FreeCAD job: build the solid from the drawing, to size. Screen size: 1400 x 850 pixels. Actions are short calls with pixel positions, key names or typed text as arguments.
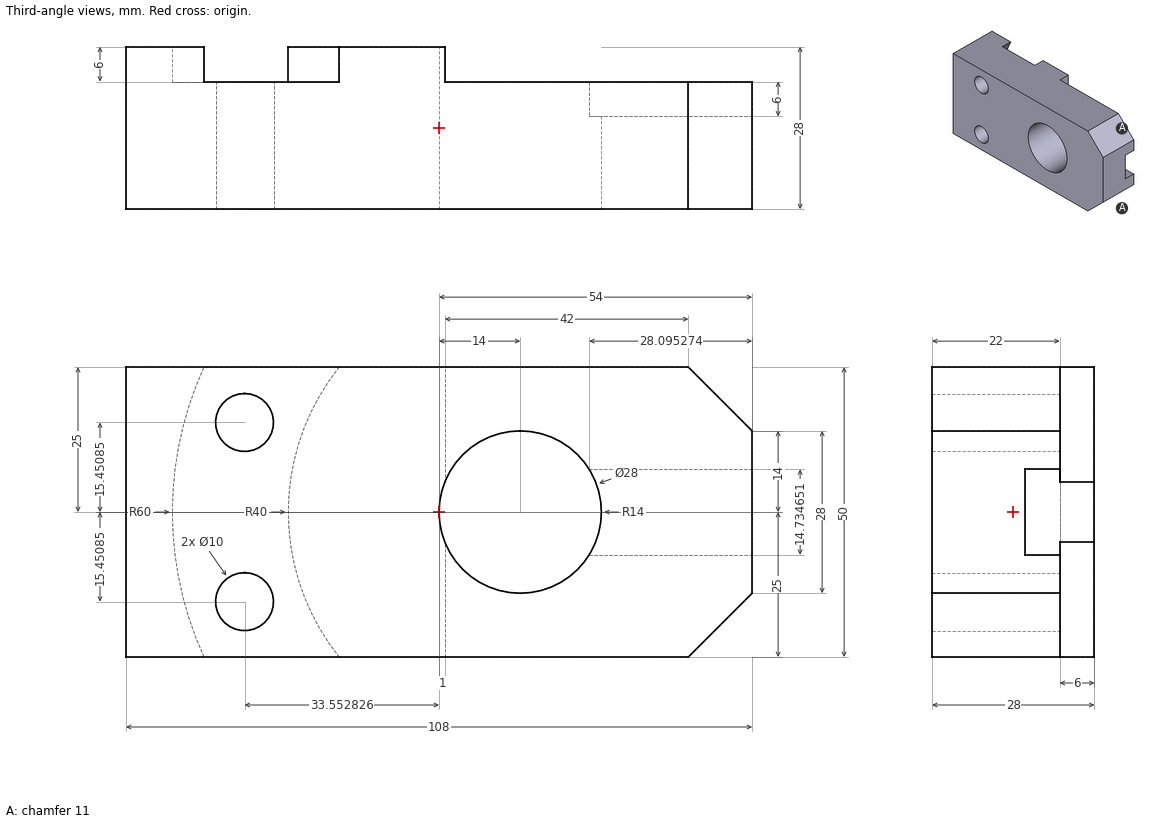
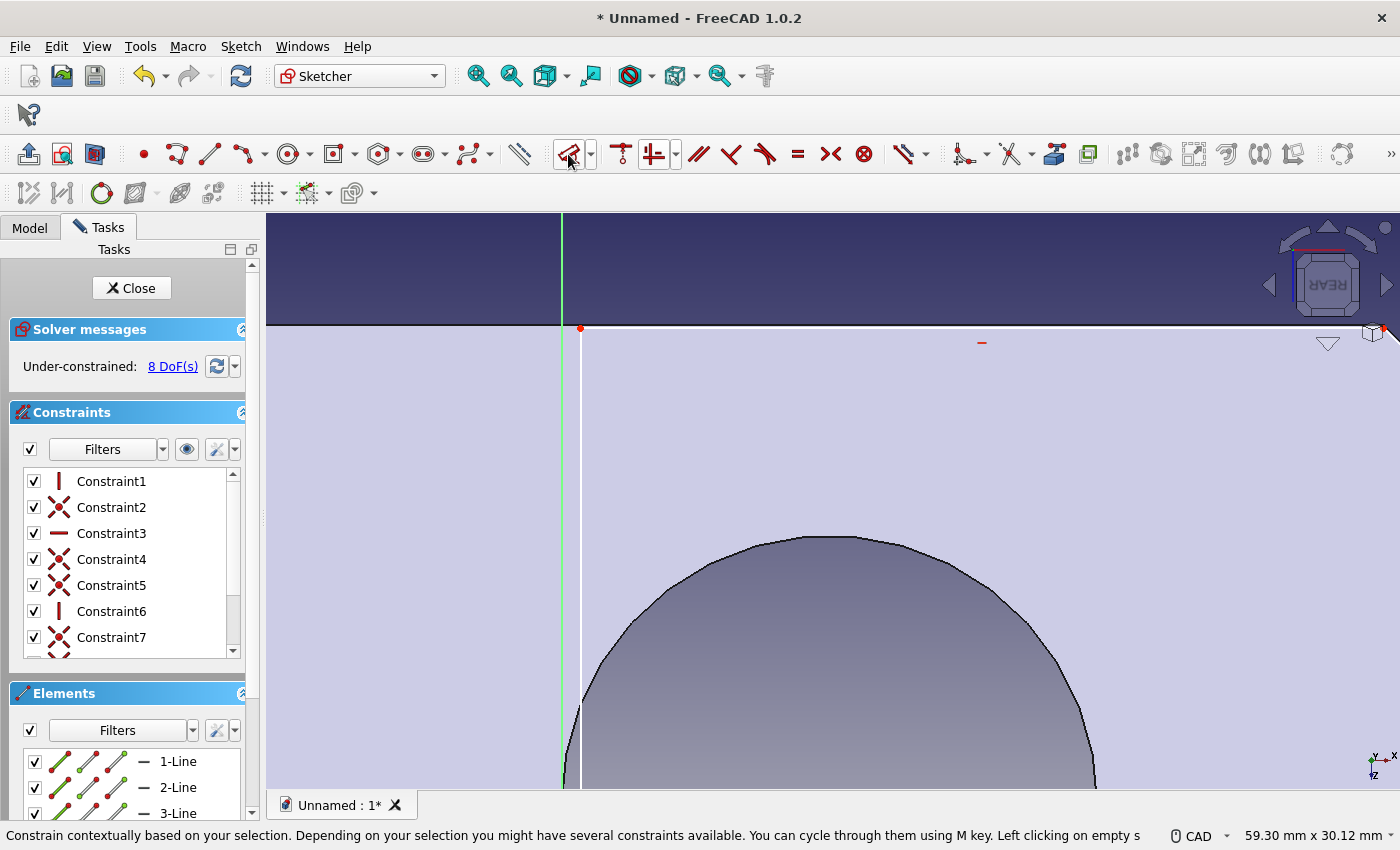
click(581, 615)
click(547, 545)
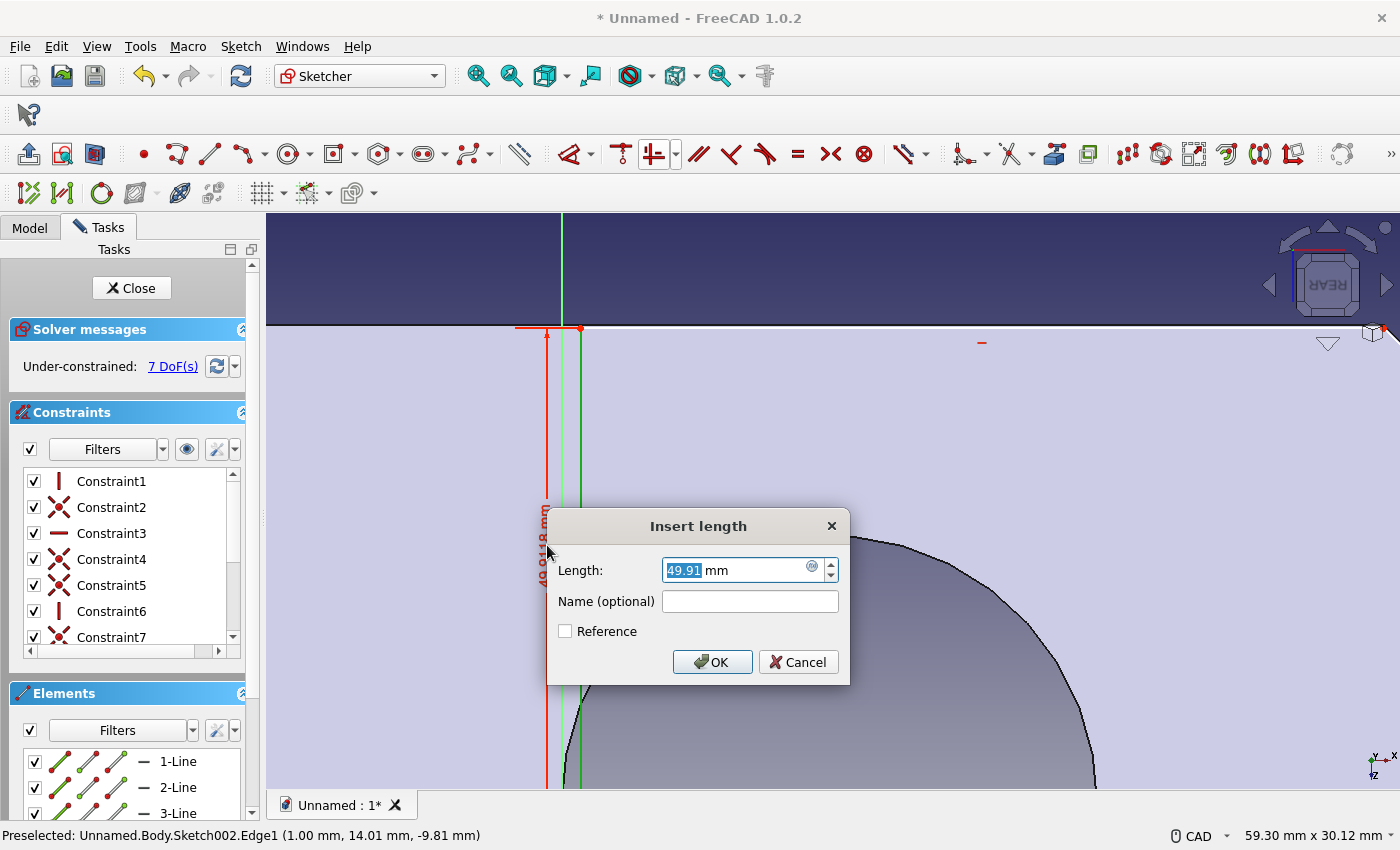
text(50)
key(Return)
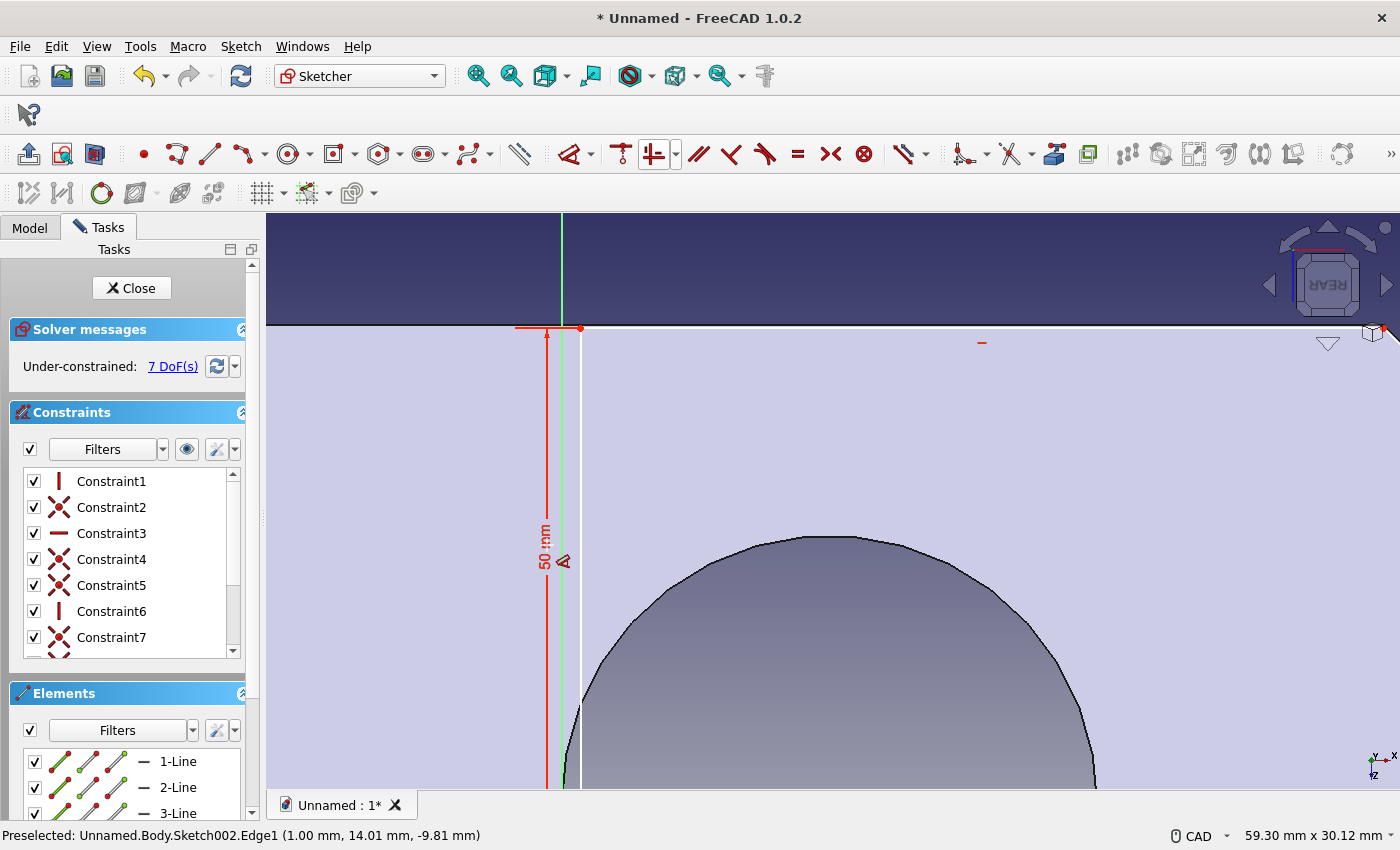
scroll(582, 325, down, 5)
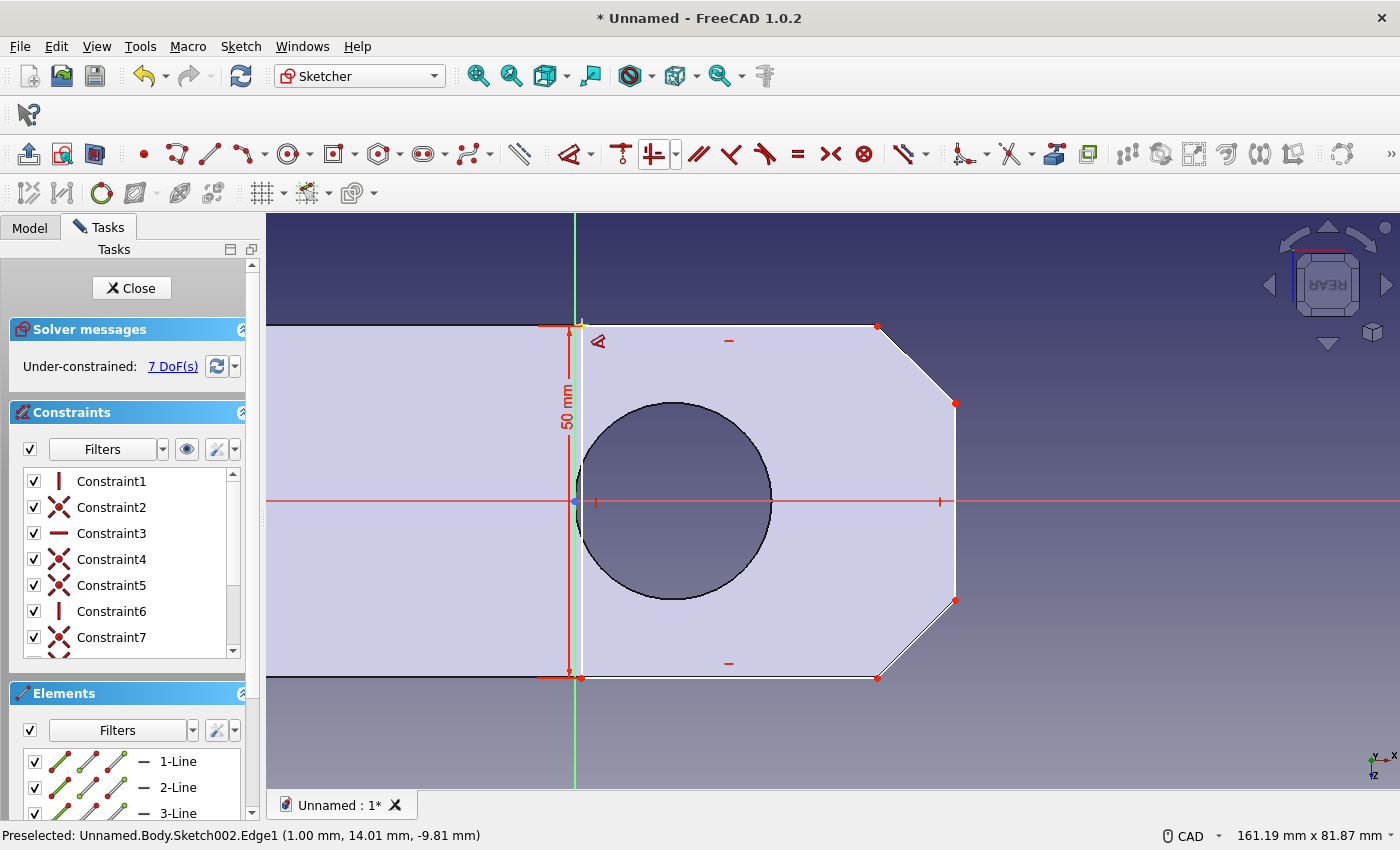
click(670, 678)
click(729, 712)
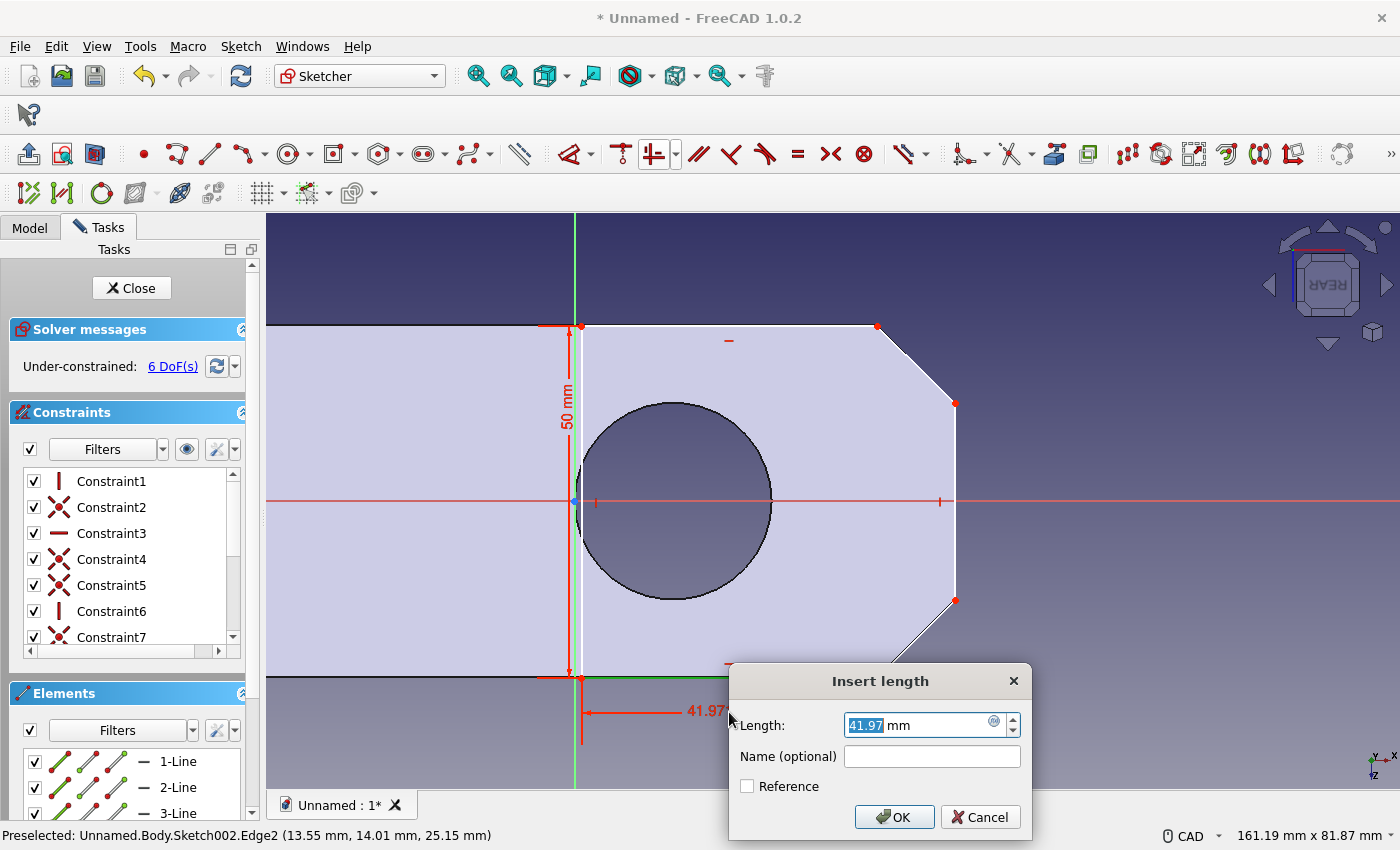
text(42)
key(Return)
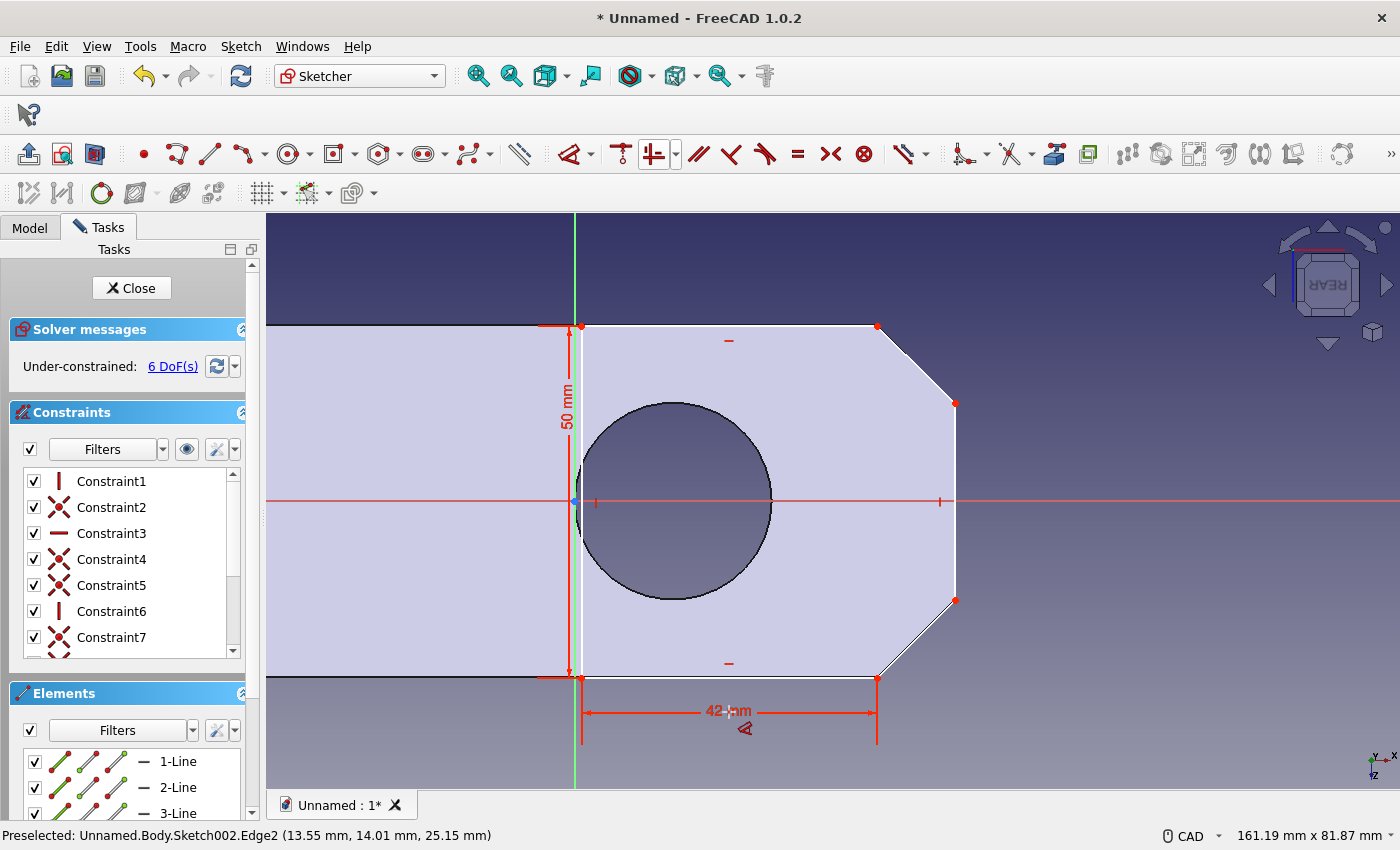
click(955, 541)
click(989, 457)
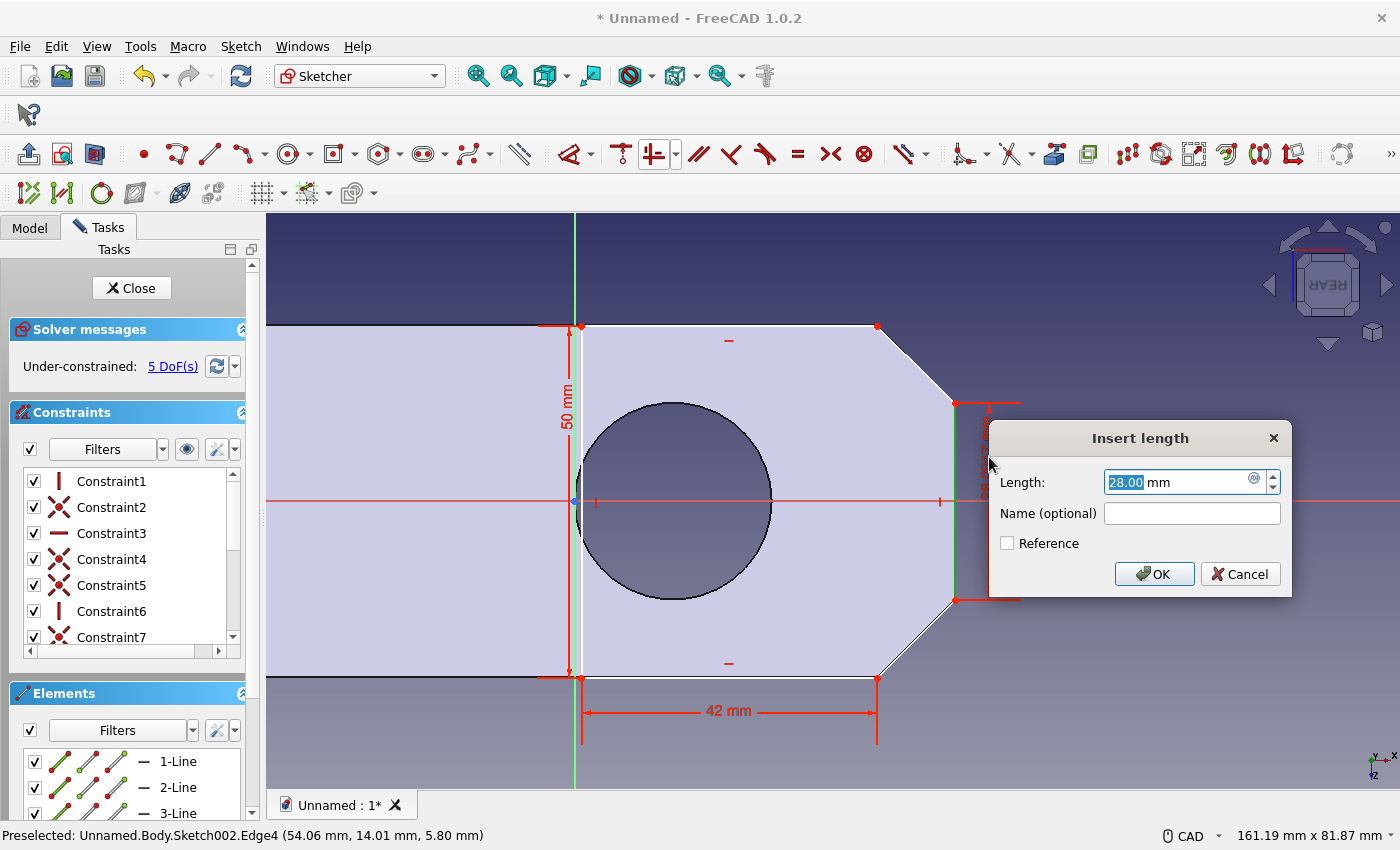
text(28)
key(Return)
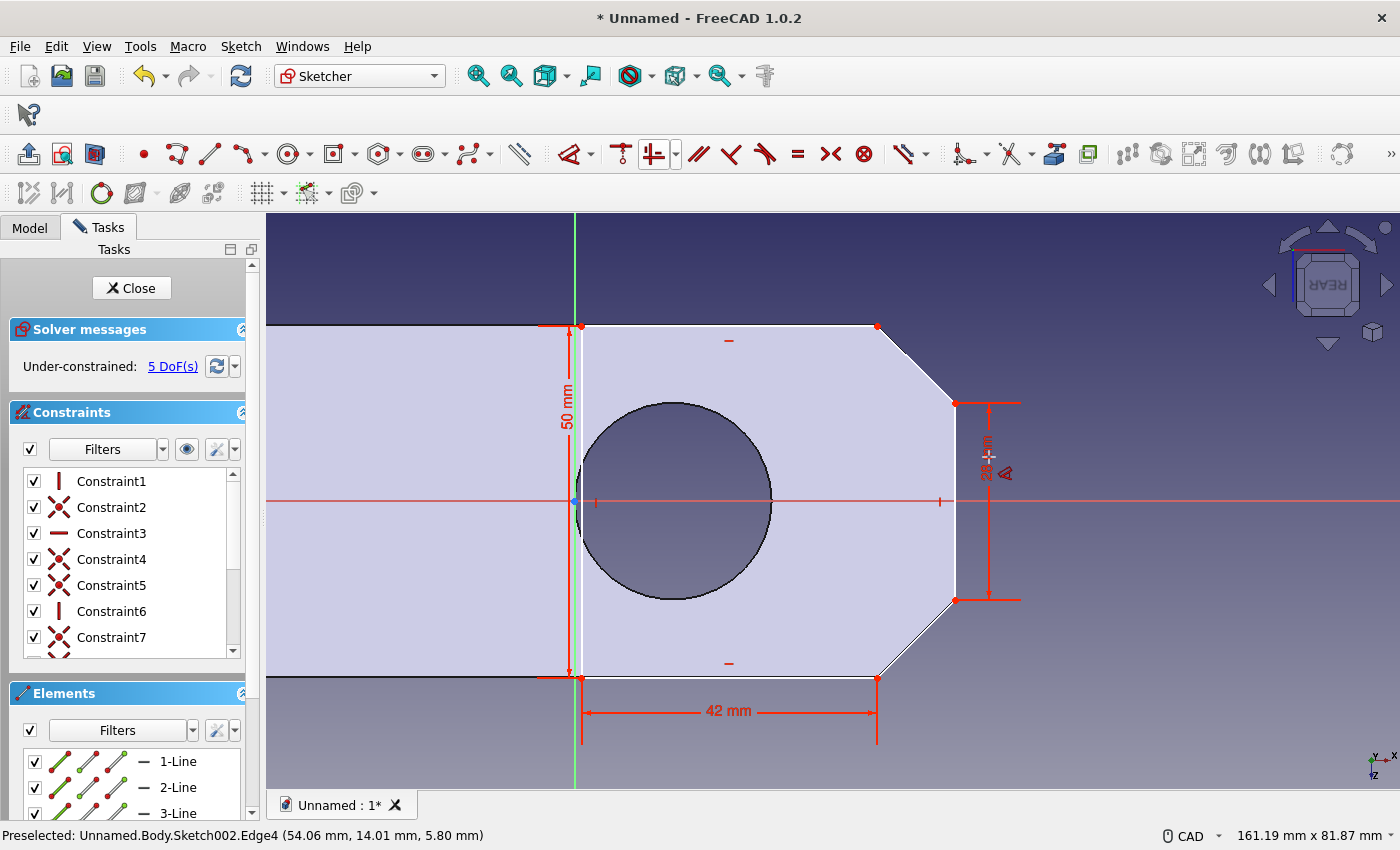
click(788, 326)
click(729, 292)